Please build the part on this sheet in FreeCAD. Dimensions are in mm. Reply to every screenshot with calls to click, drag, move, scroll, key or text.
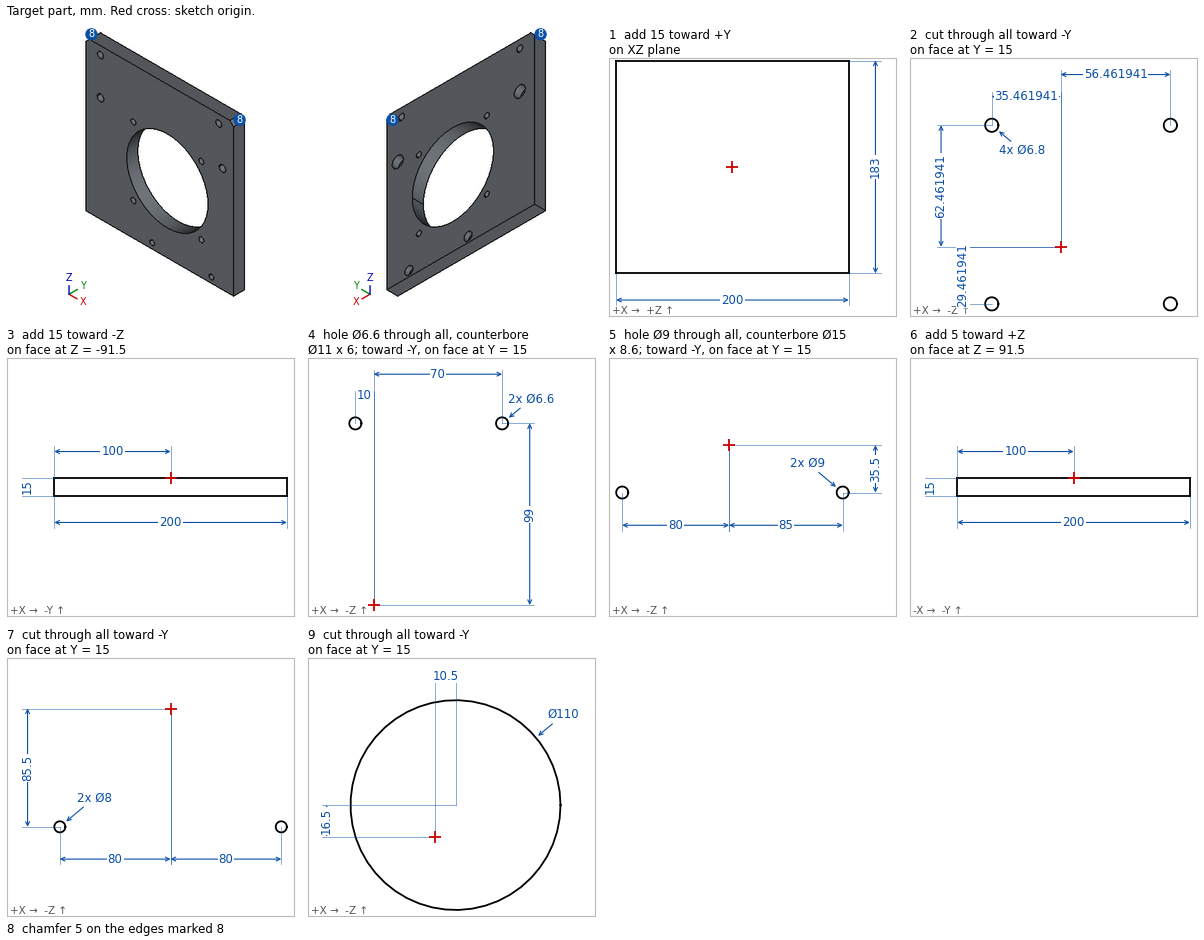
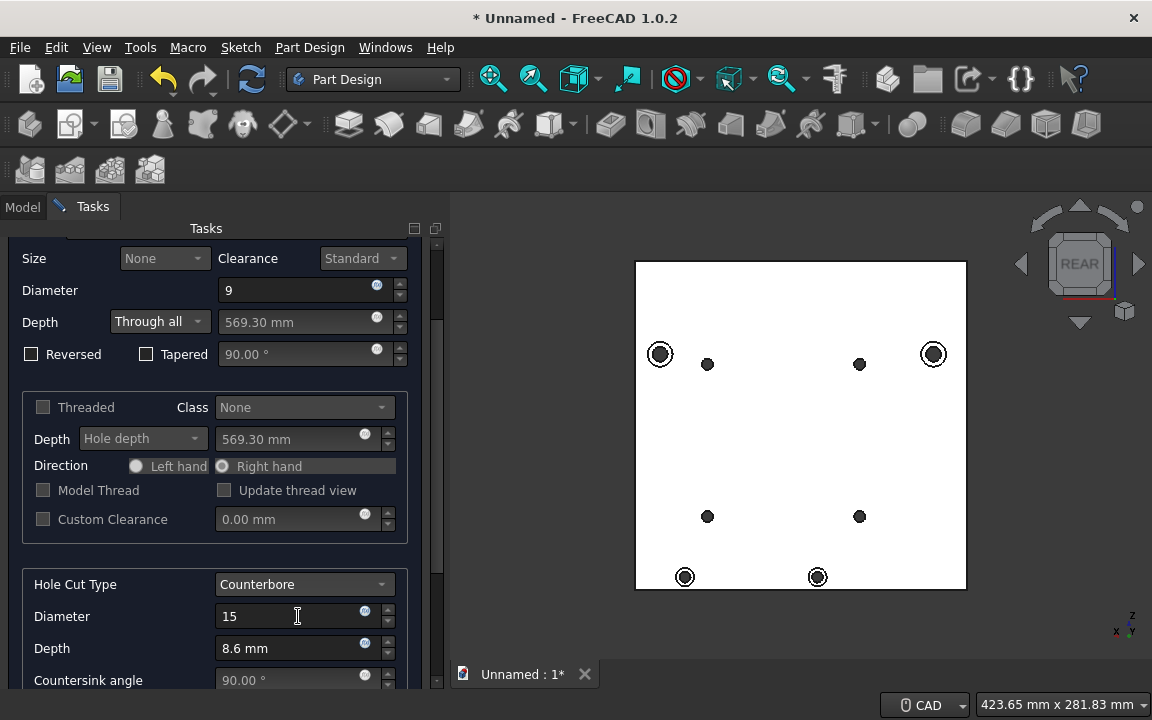
scroll(437, 463, up, 3)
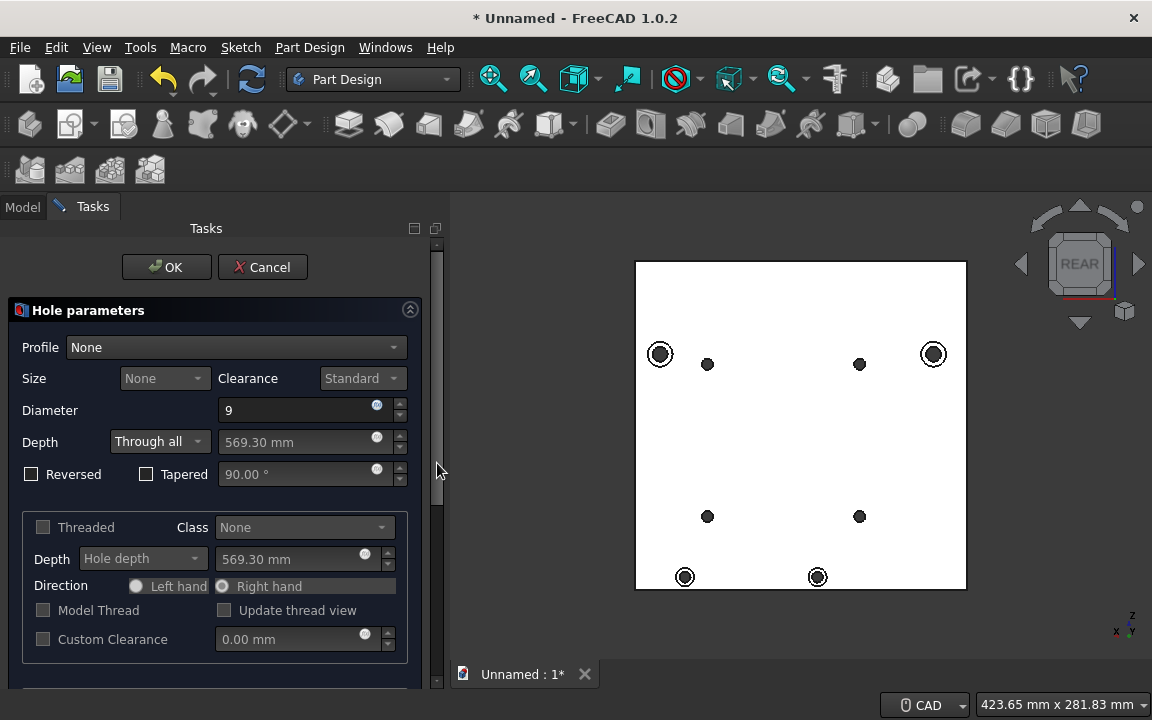
click(167, 267)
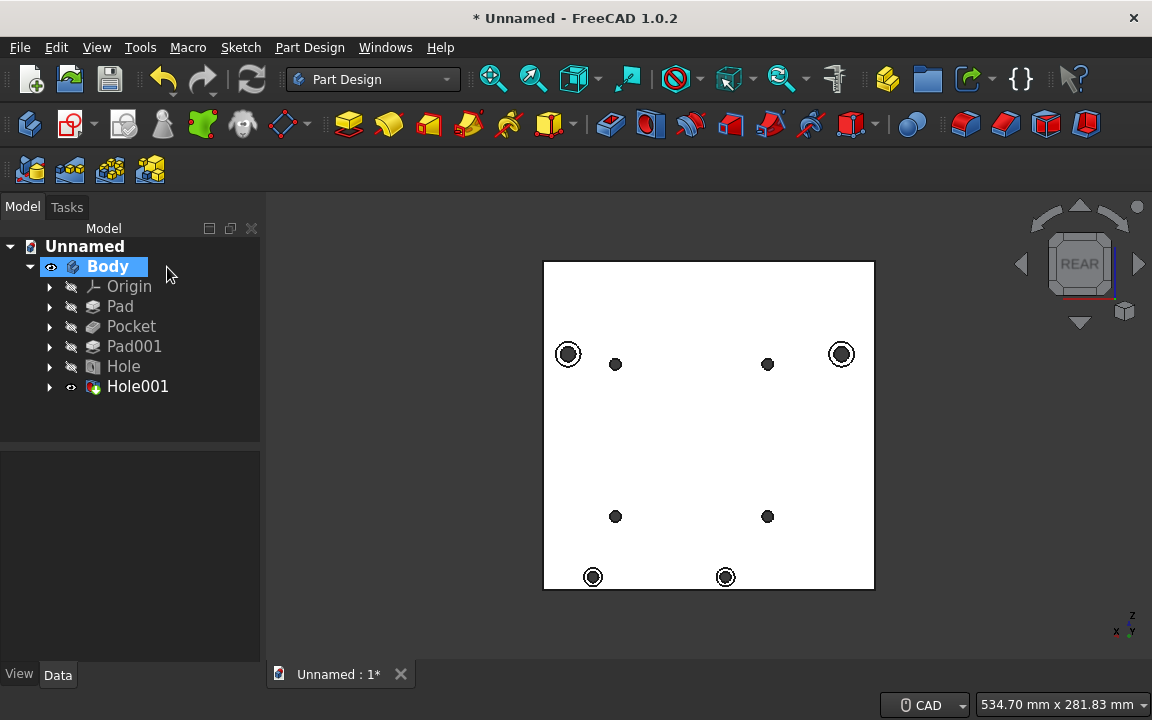
key(0)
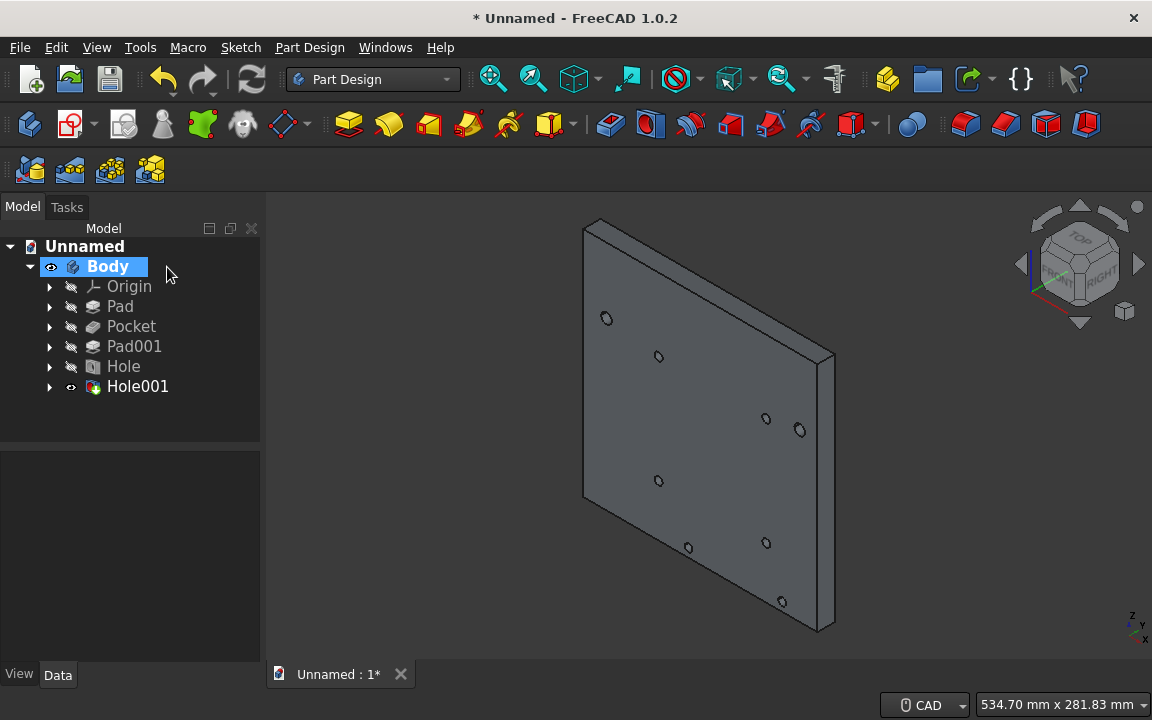
click(676, 271)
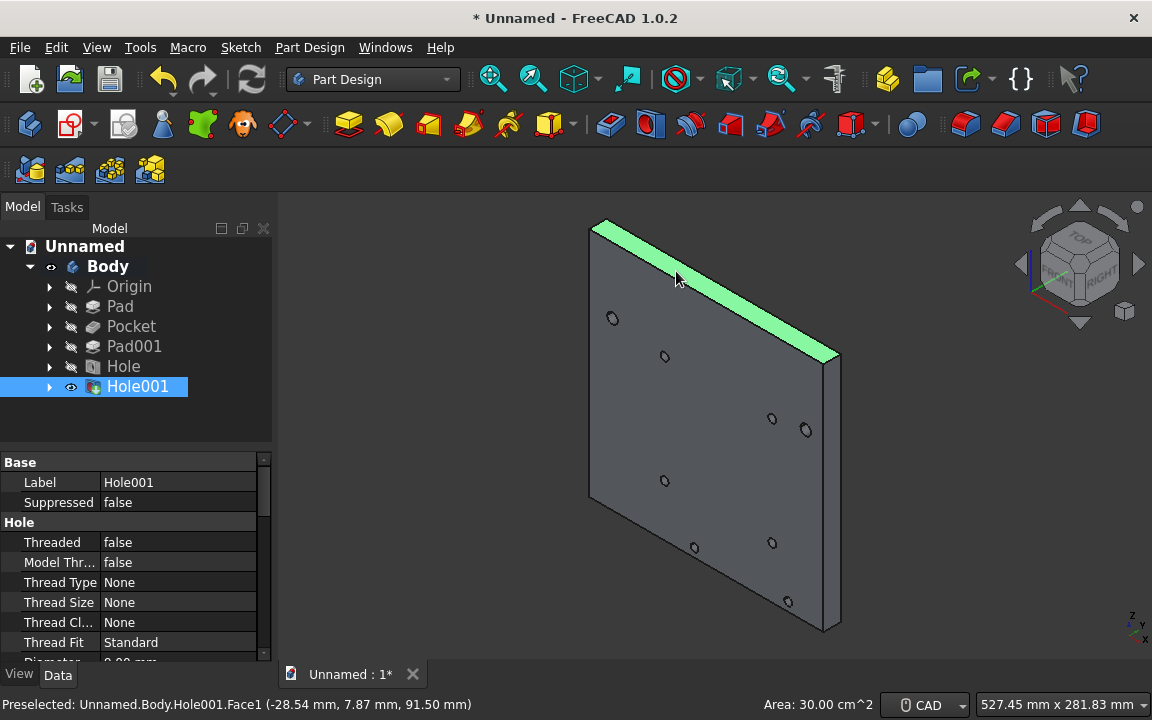
click(70, 124)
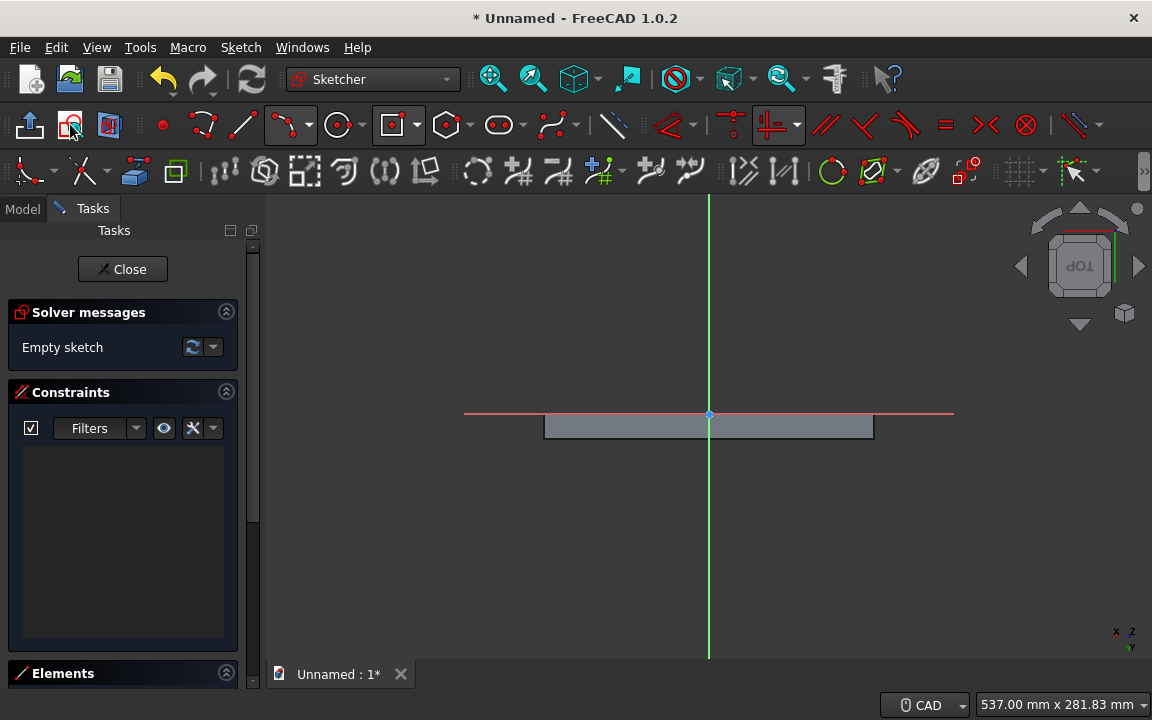
scroll(848, 427, up, 2)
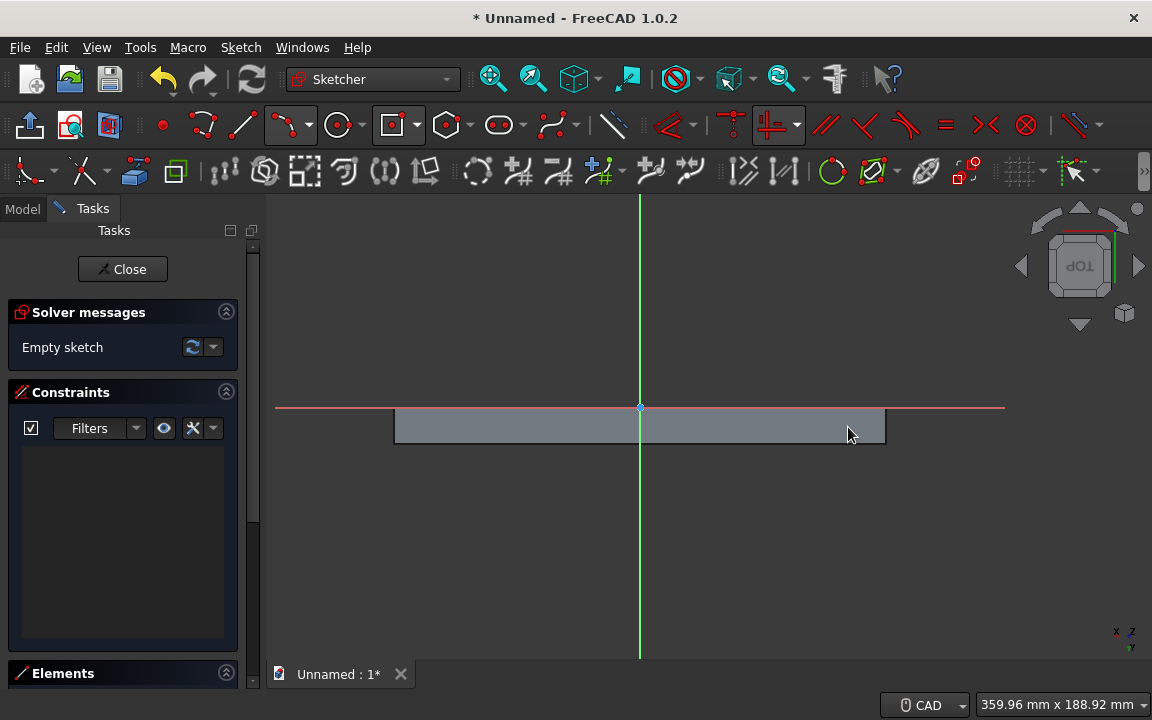
click(420, 126)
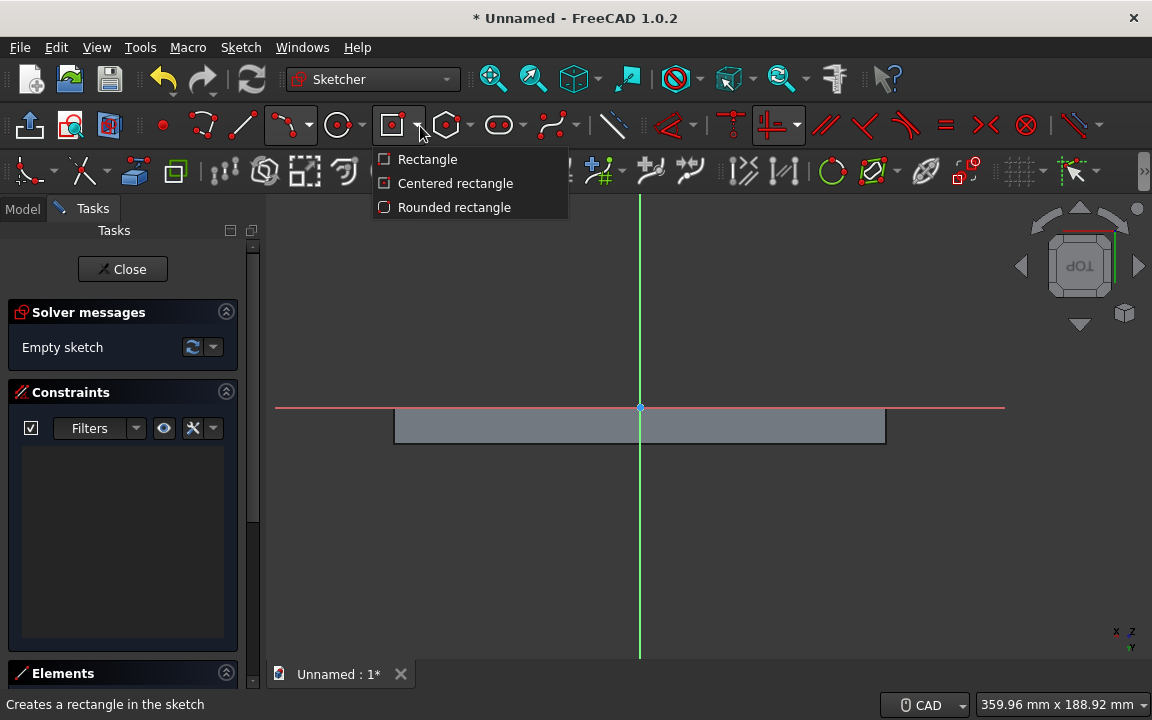
click(470, 159)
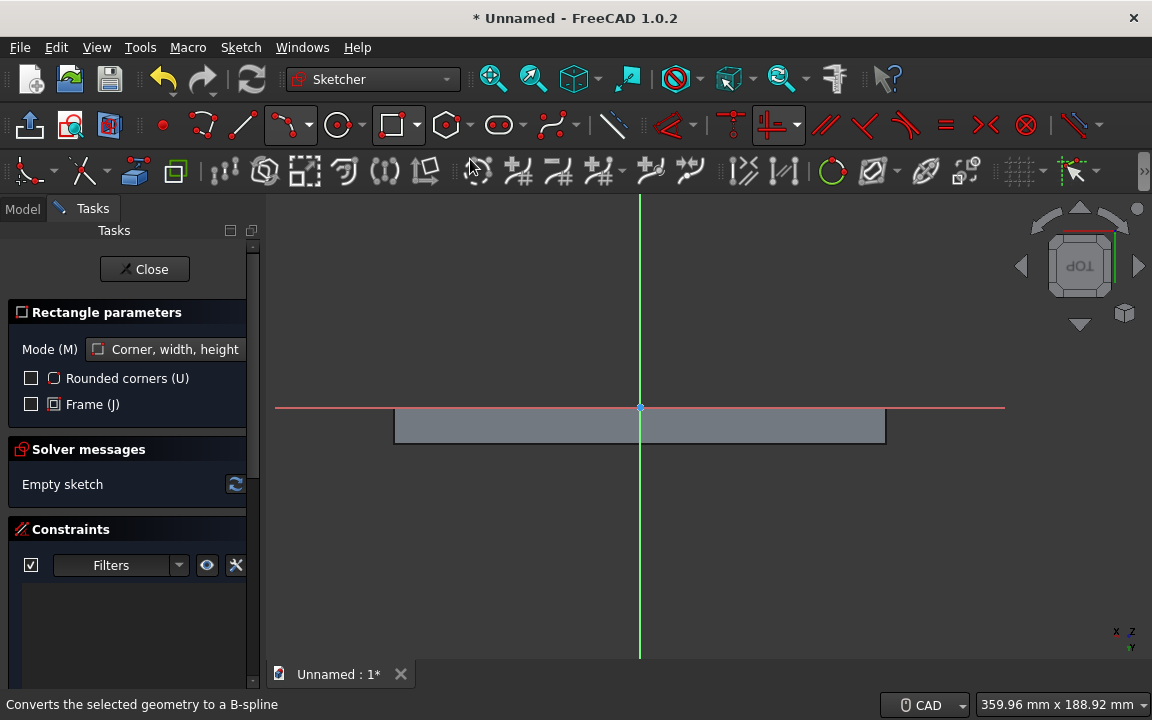
click(394, 408)
click(886, 444)
key(Escape)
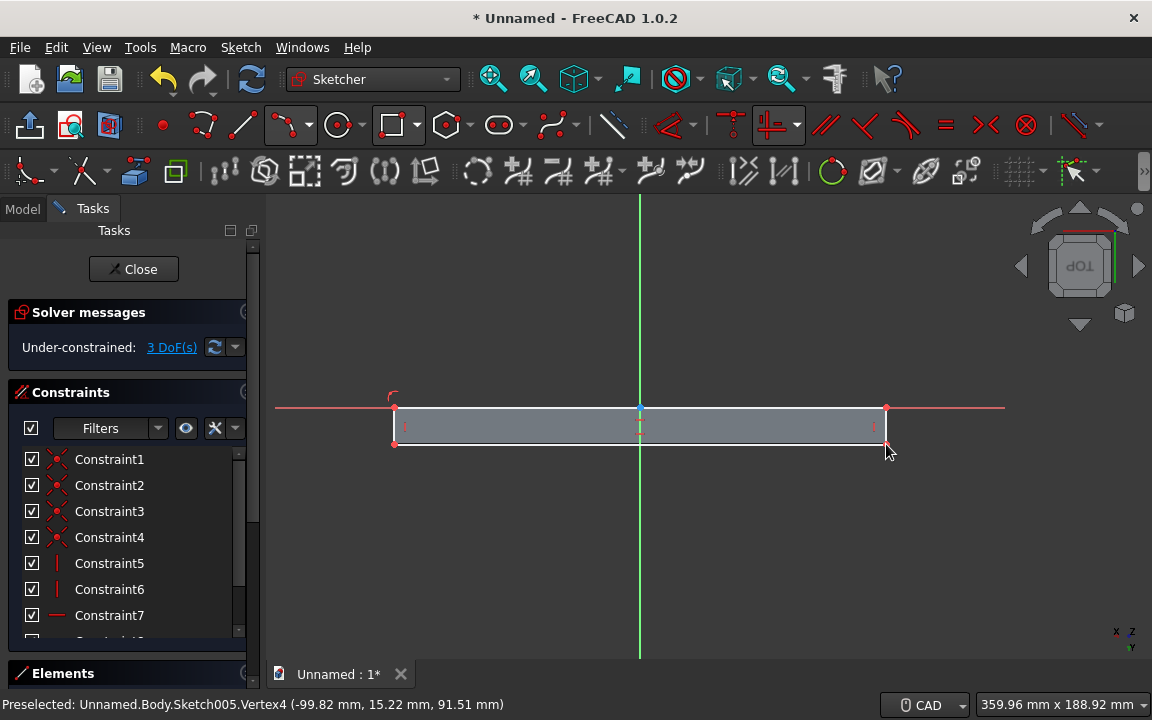
click(668, 126)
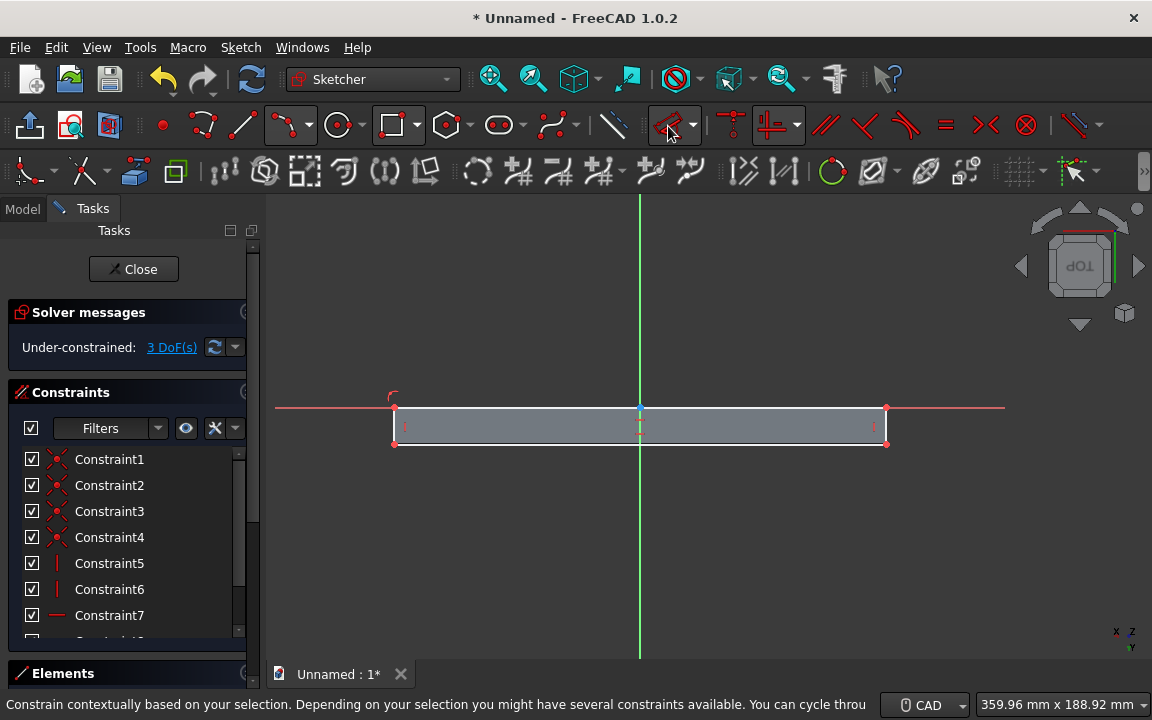
scroll(394, 419, up, 2)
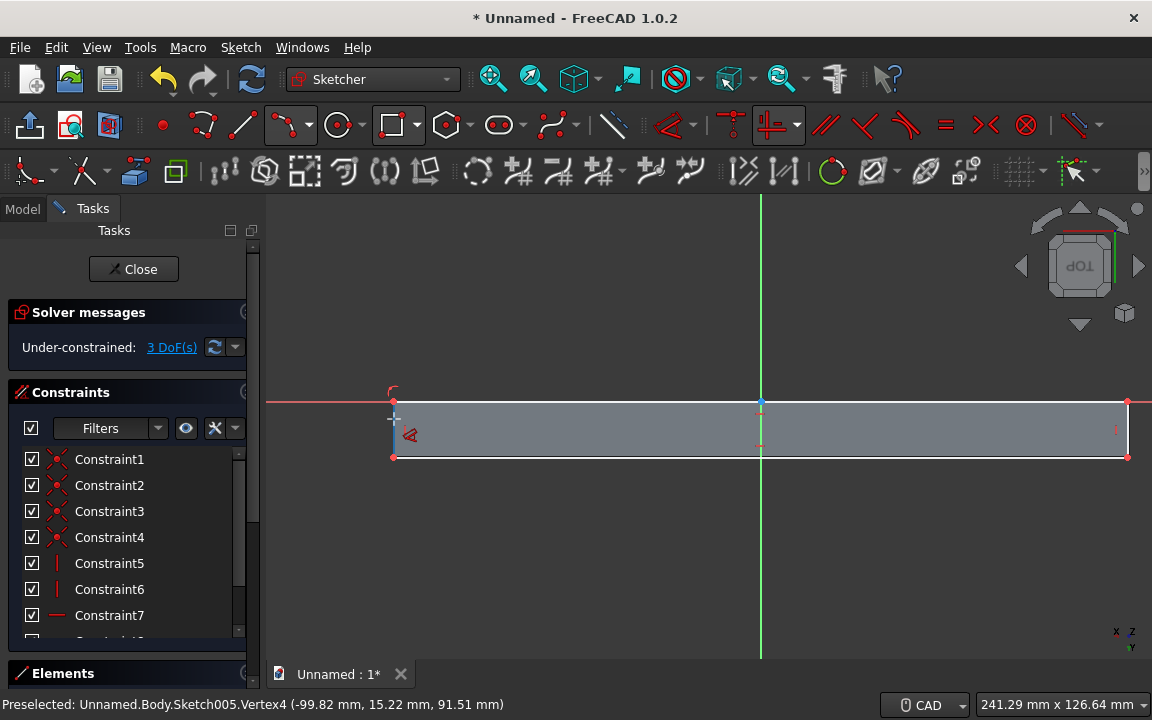
click(394, 418)
click(360, 430)